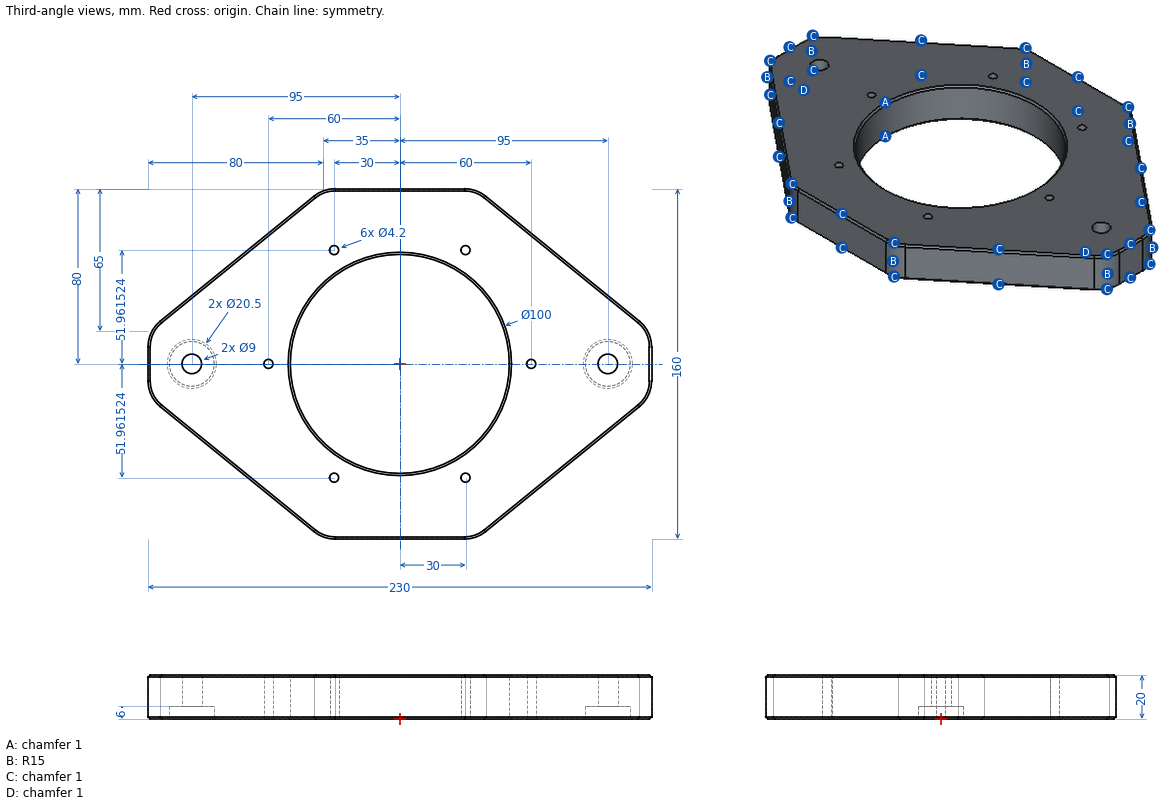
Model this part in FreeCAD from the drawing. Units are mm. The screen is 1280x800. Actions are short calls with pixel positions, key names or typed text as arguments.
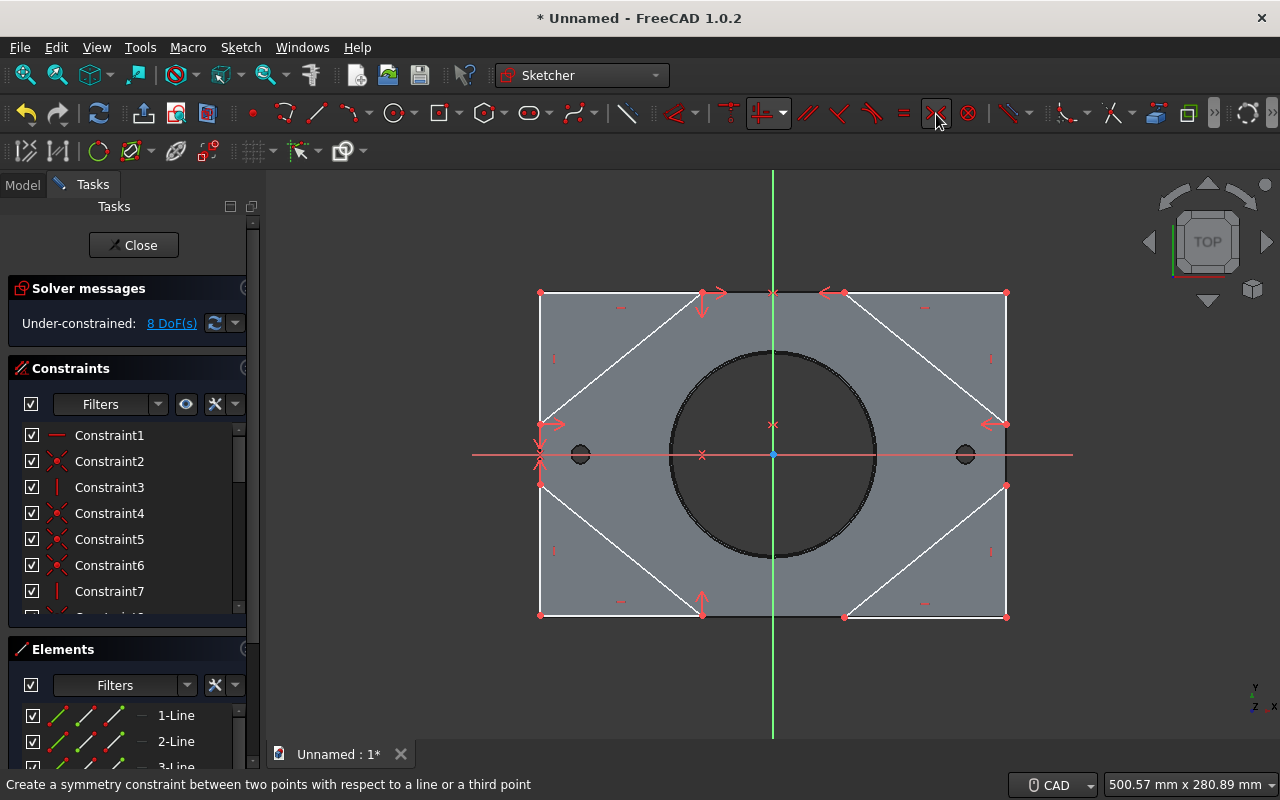
click(844, 293)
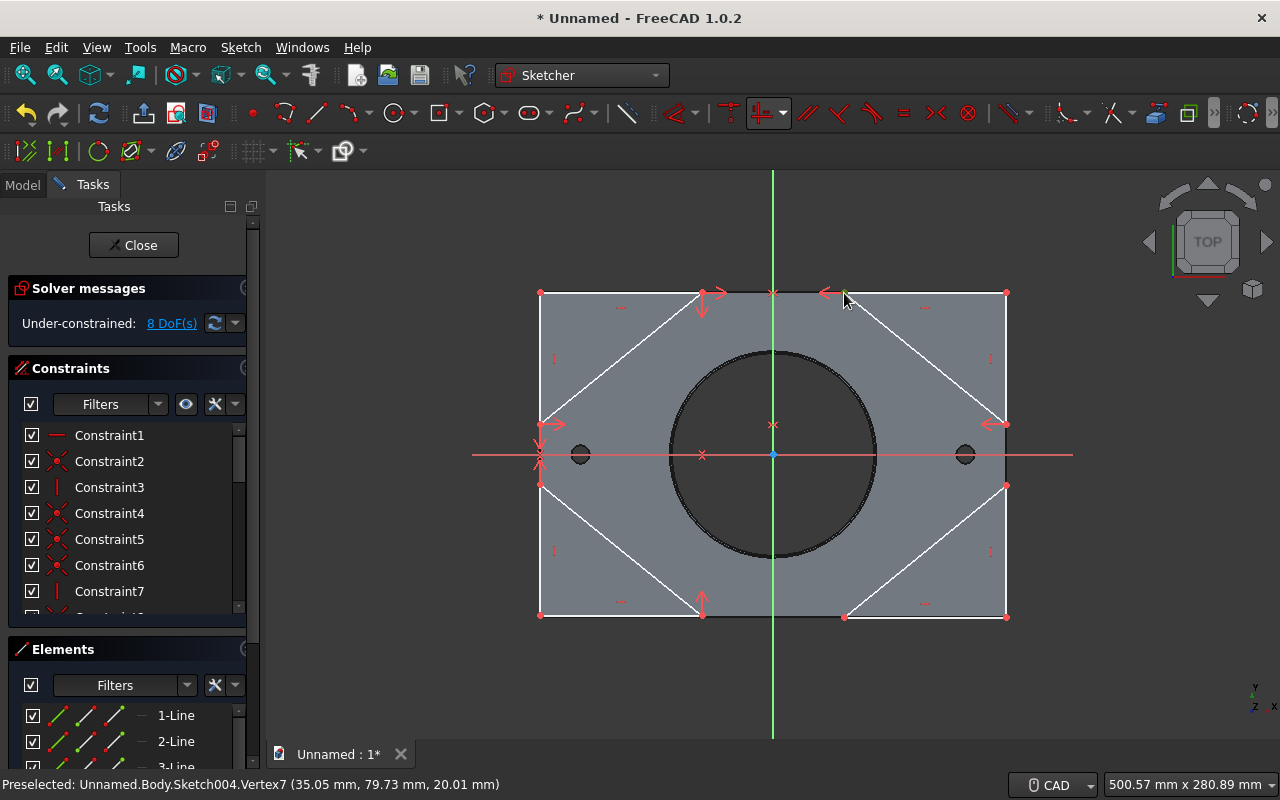
click(844, 618)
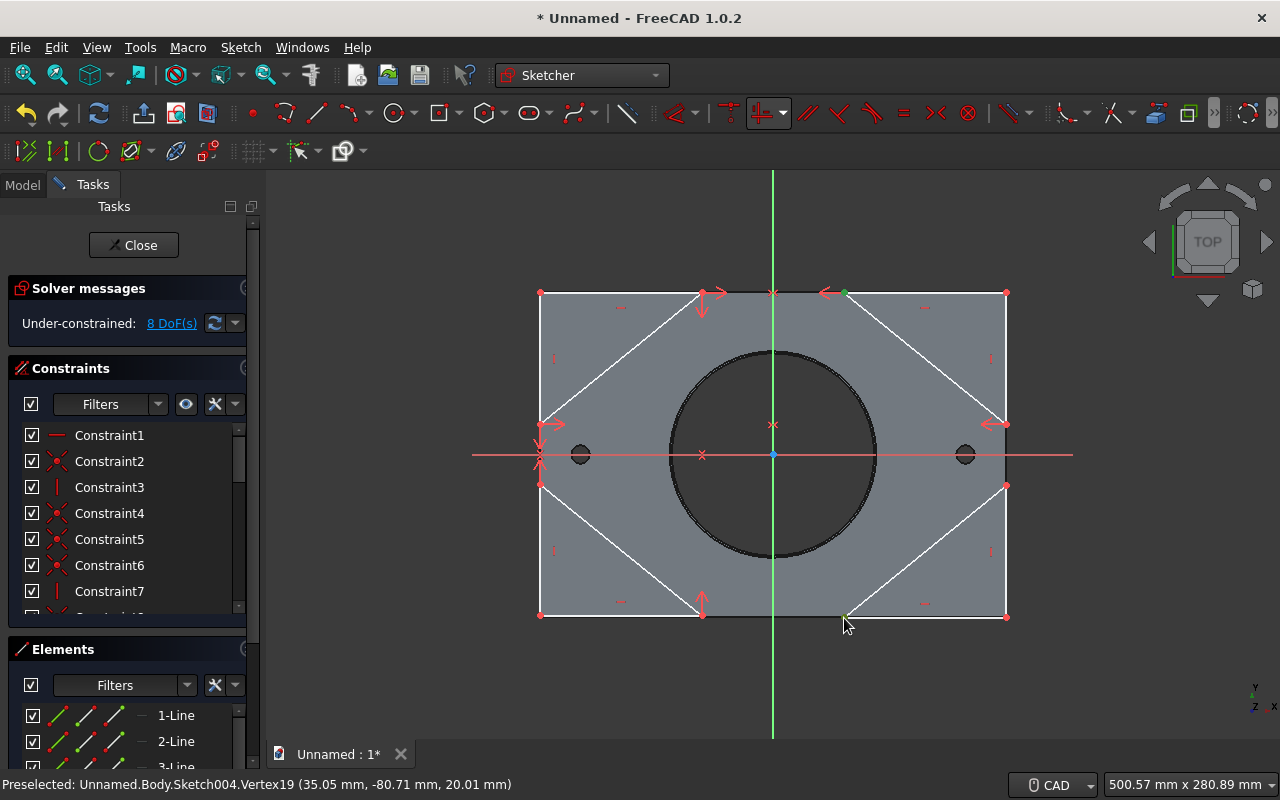
click(470, 454)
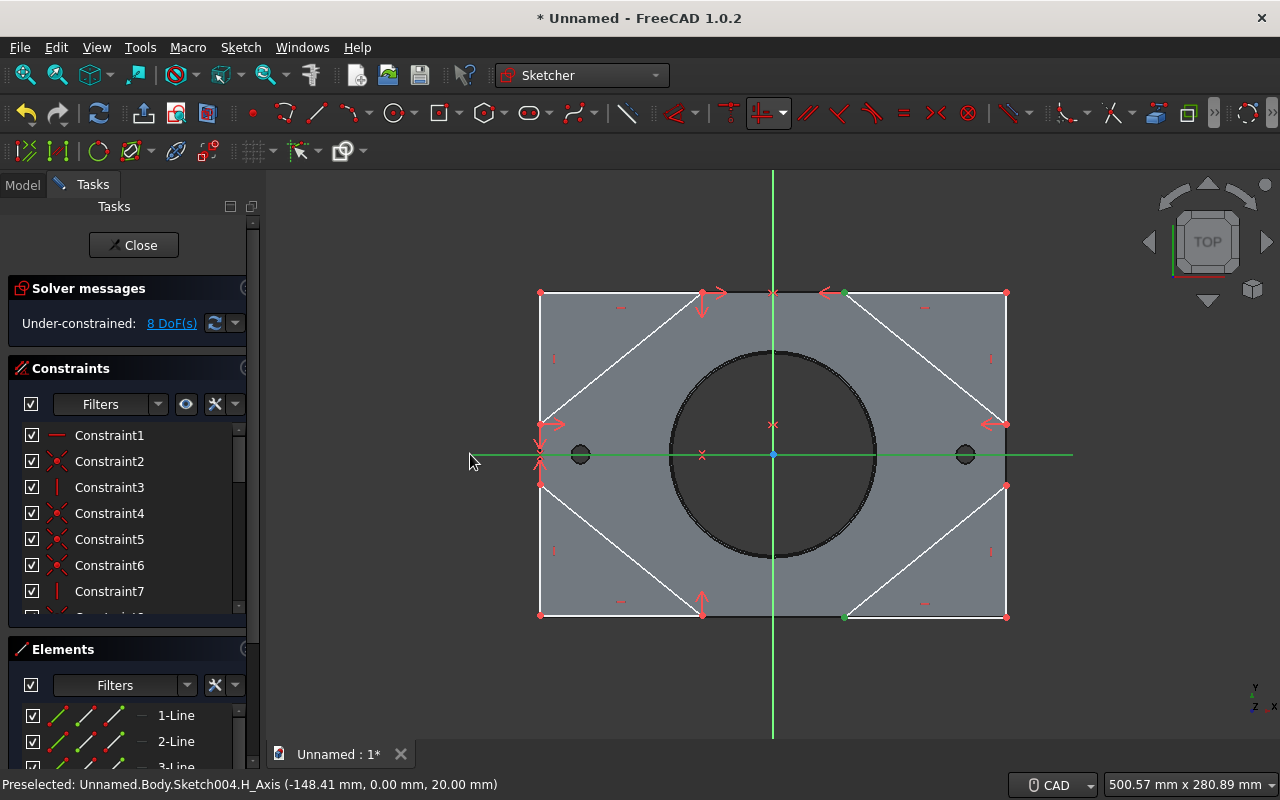
click(936, 114)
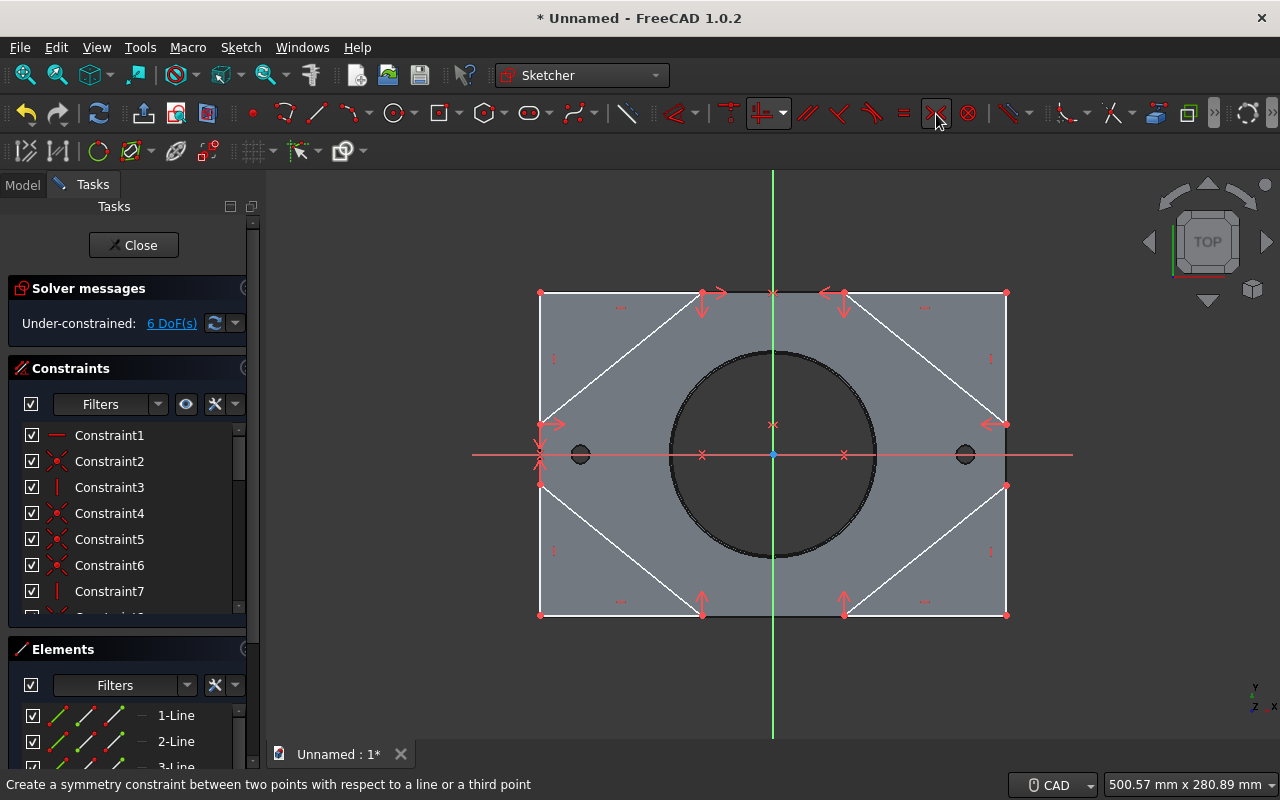
click(1006, 424)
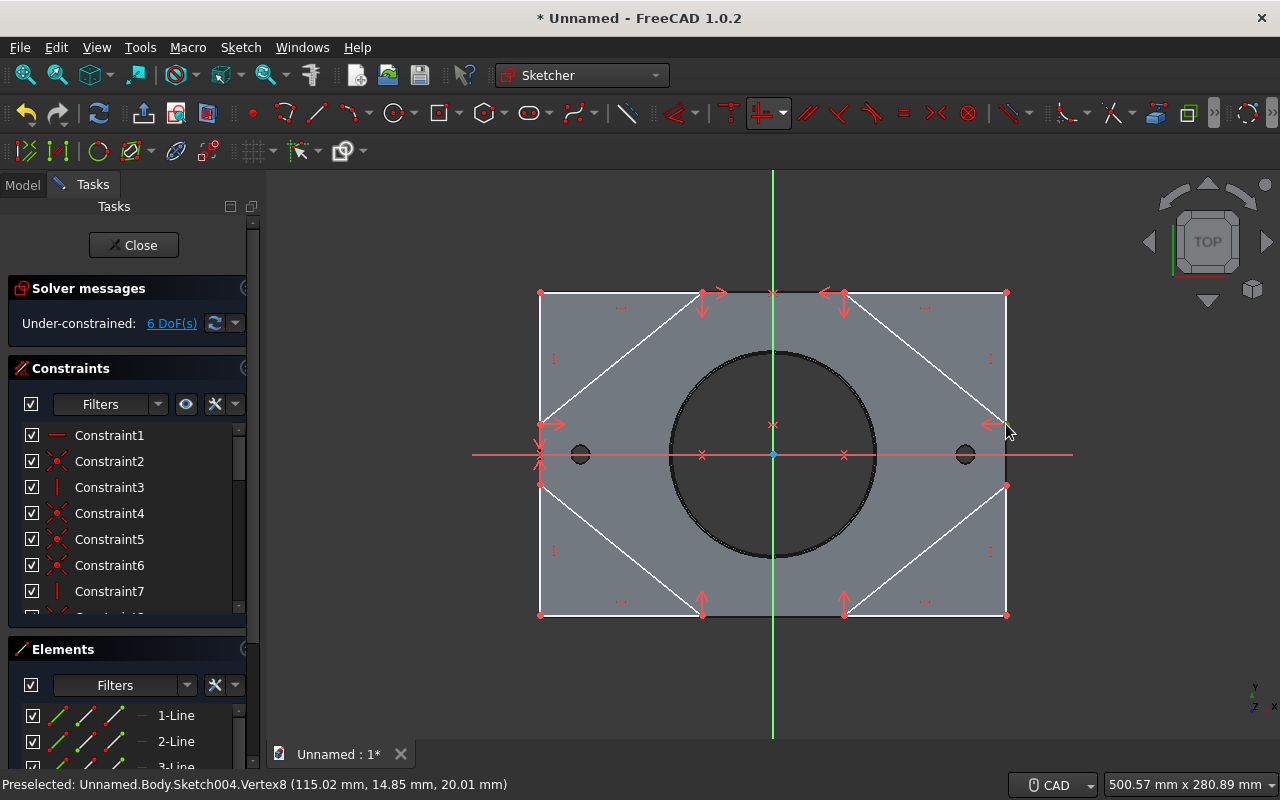
click(1006, 486)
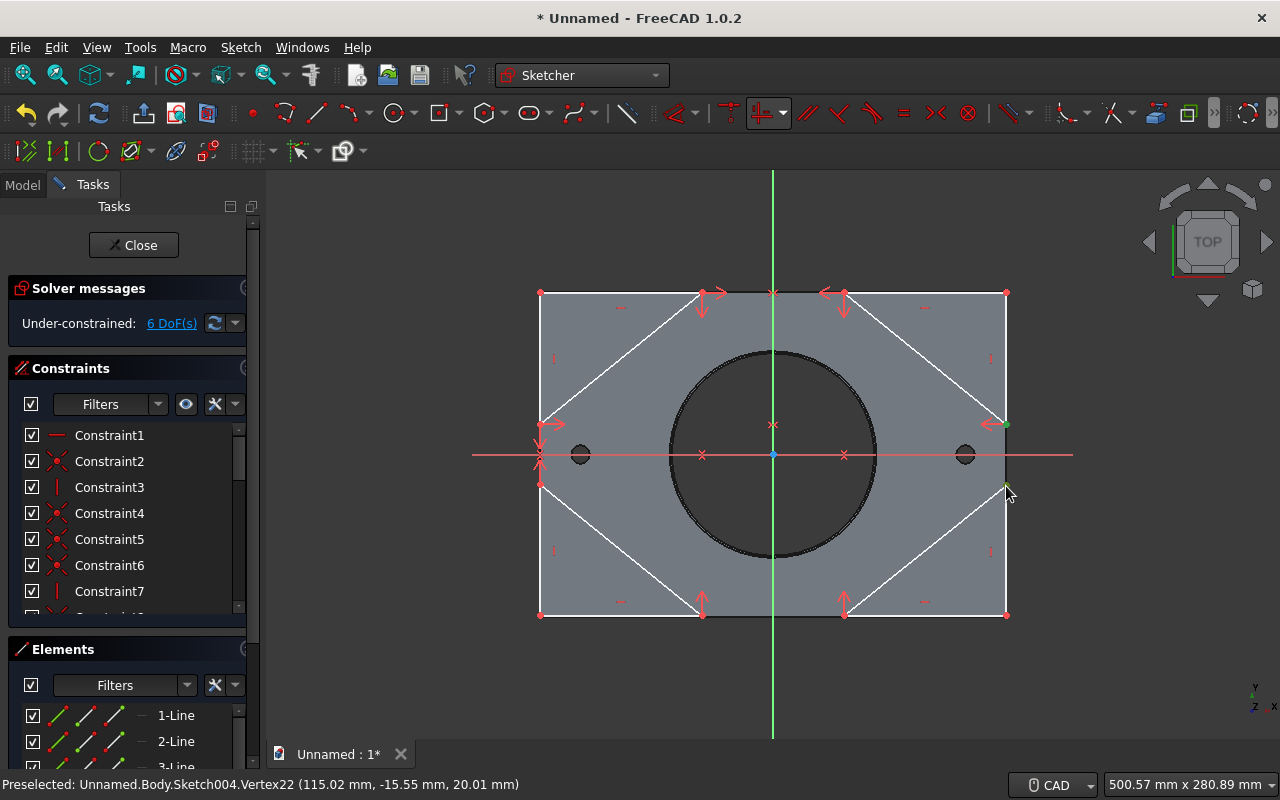
click(470, 454)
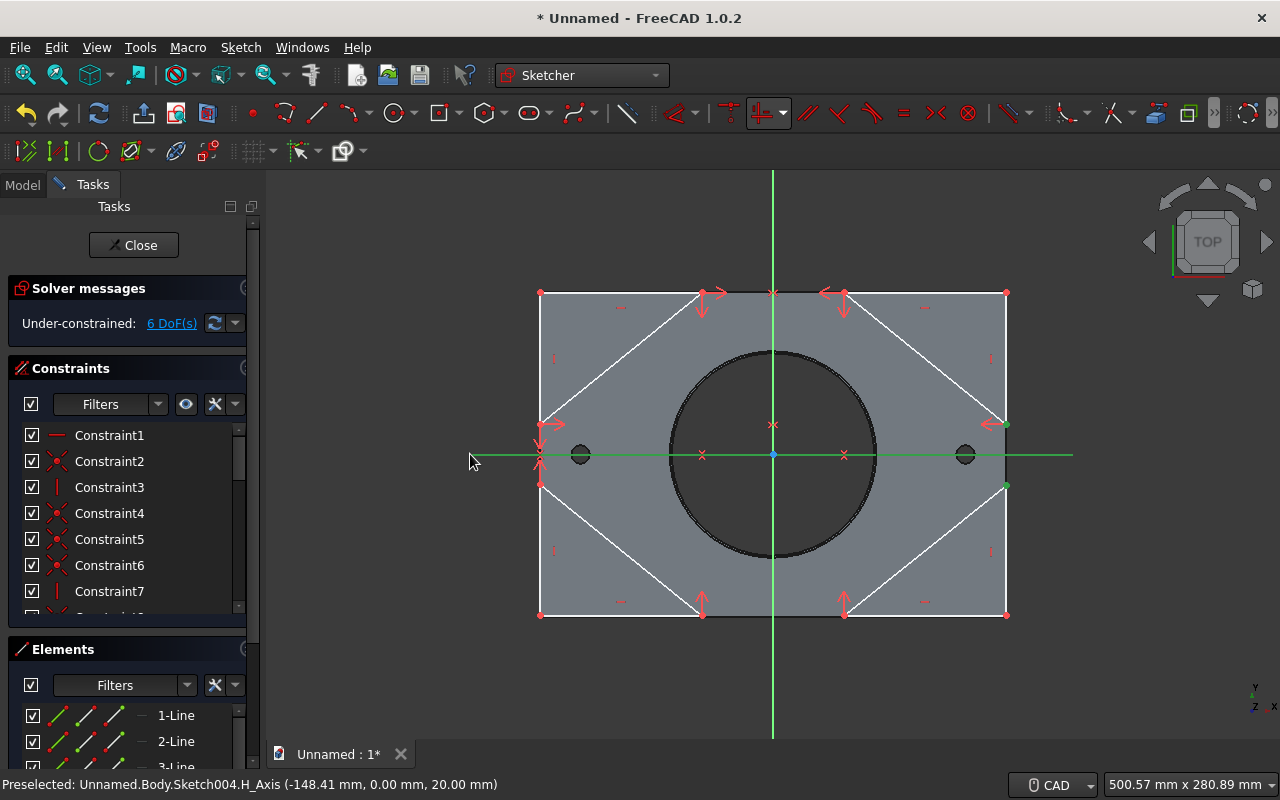
click(936, 114)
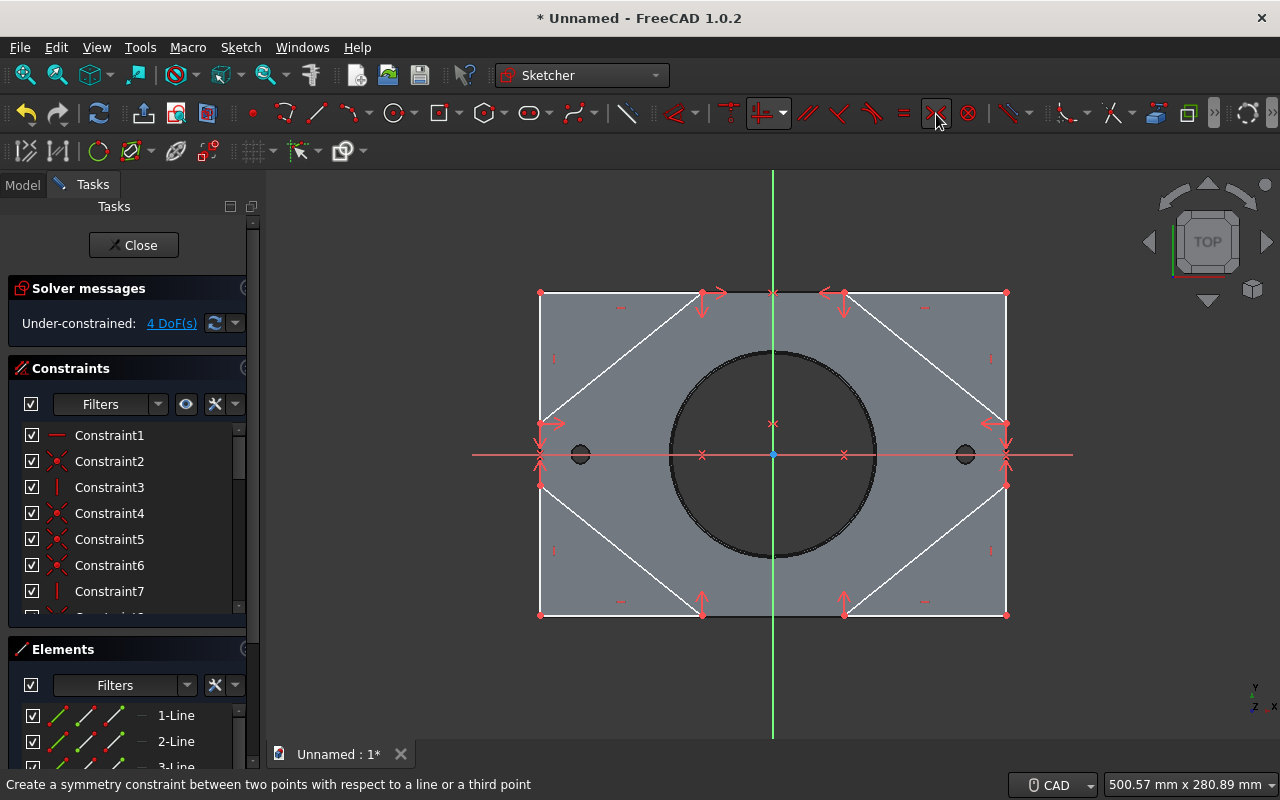
click(674, 114)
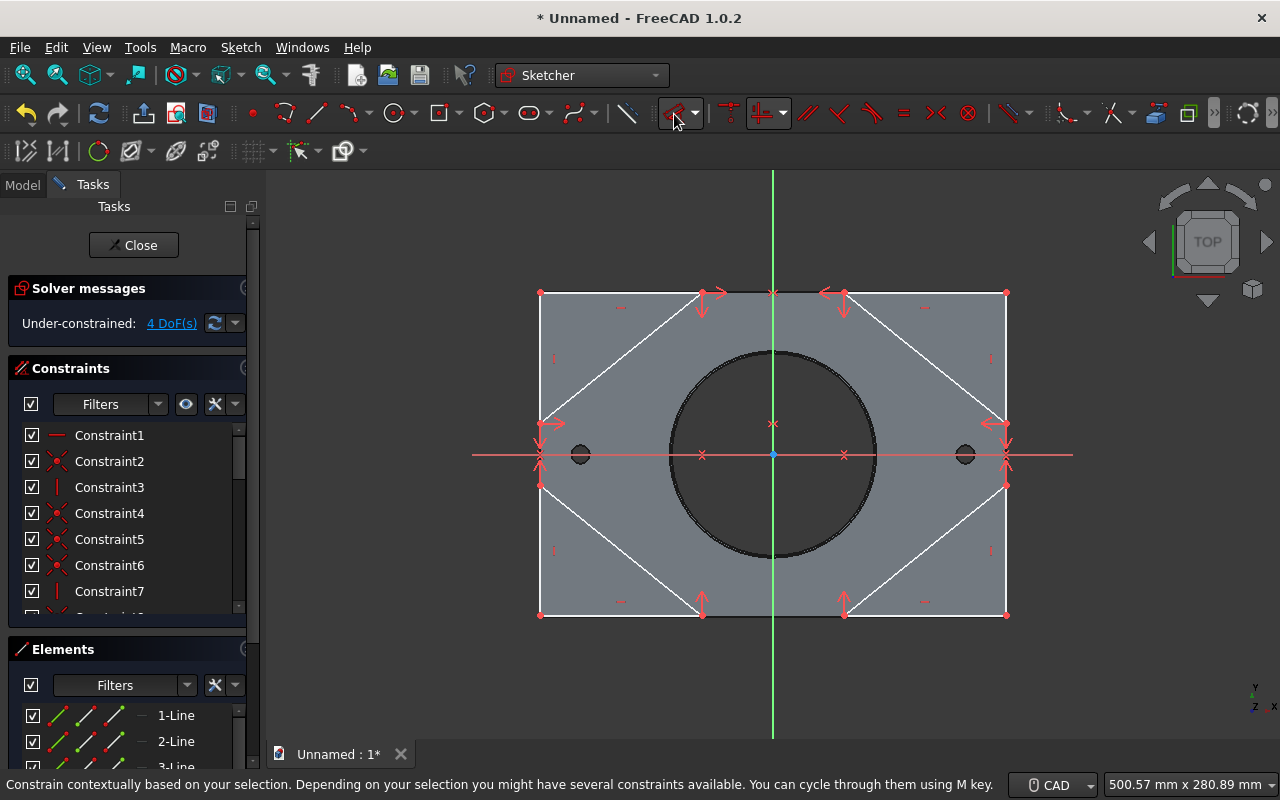
click(653, 293)
click(621, 259)